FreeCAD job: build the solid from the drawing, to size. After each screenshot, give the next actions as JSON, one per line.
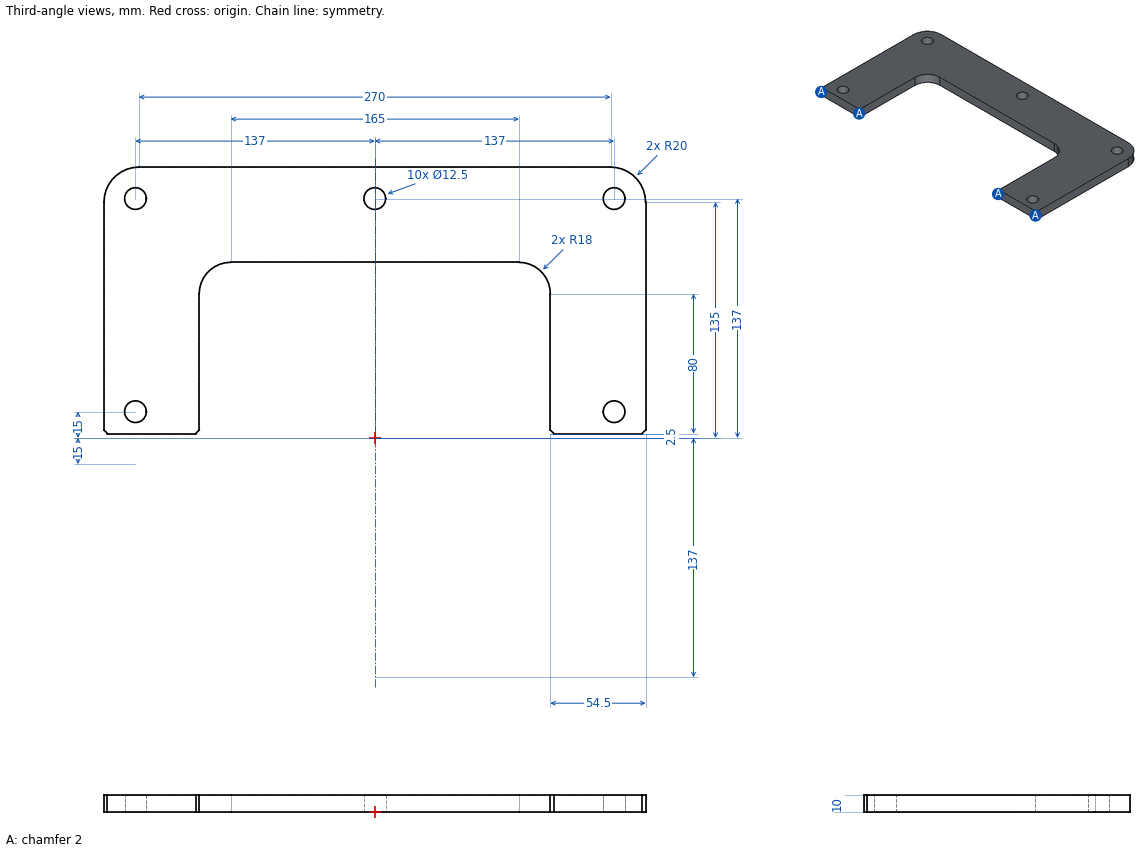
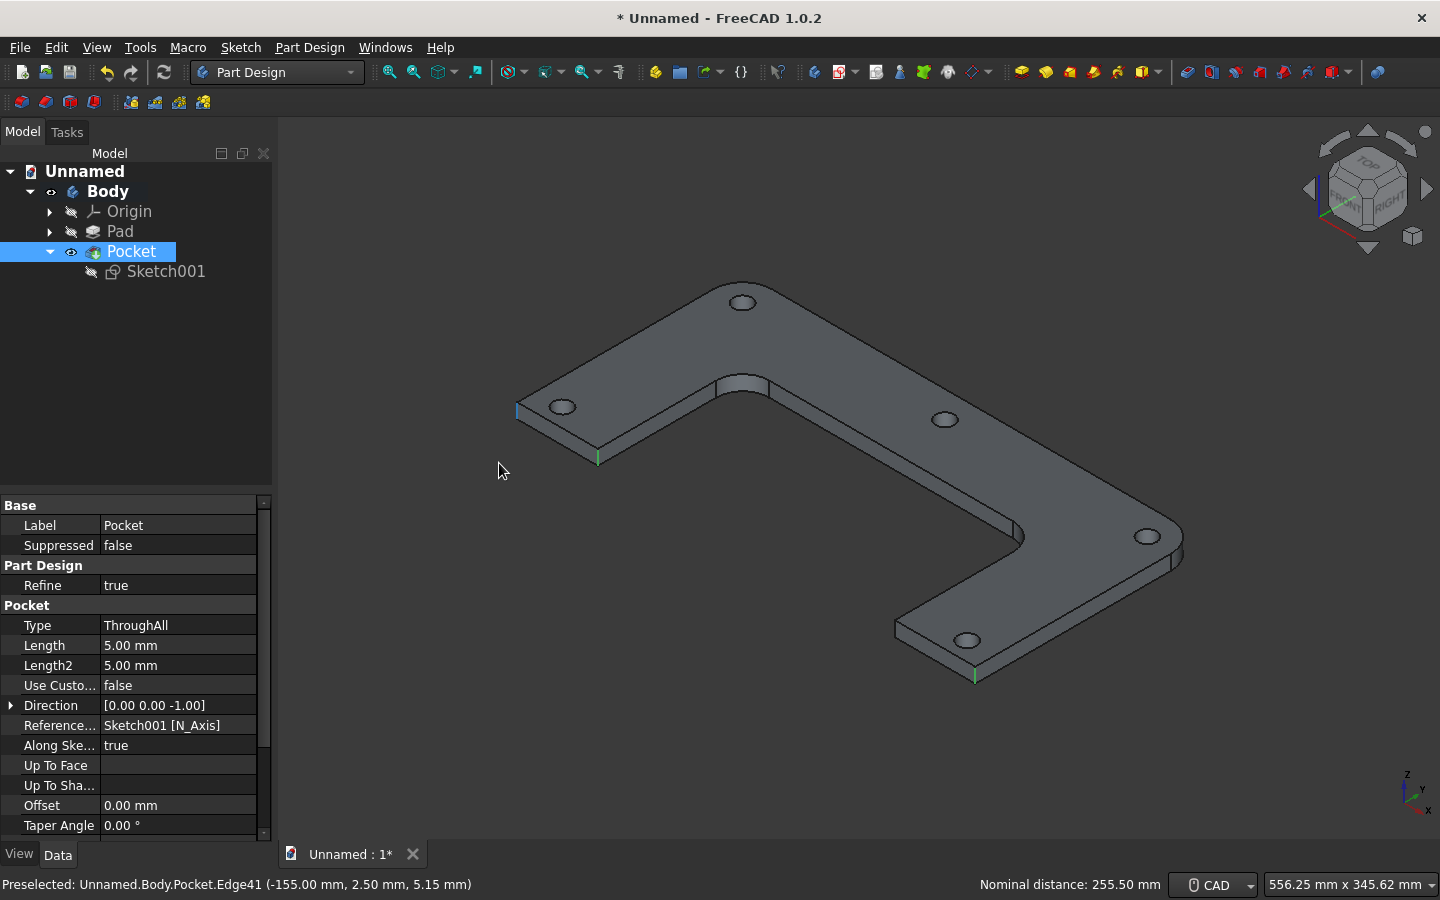
{"action": "scroll", "coordinate": [517, 410], "scroll_direction": "up", "scroll_amount": 4}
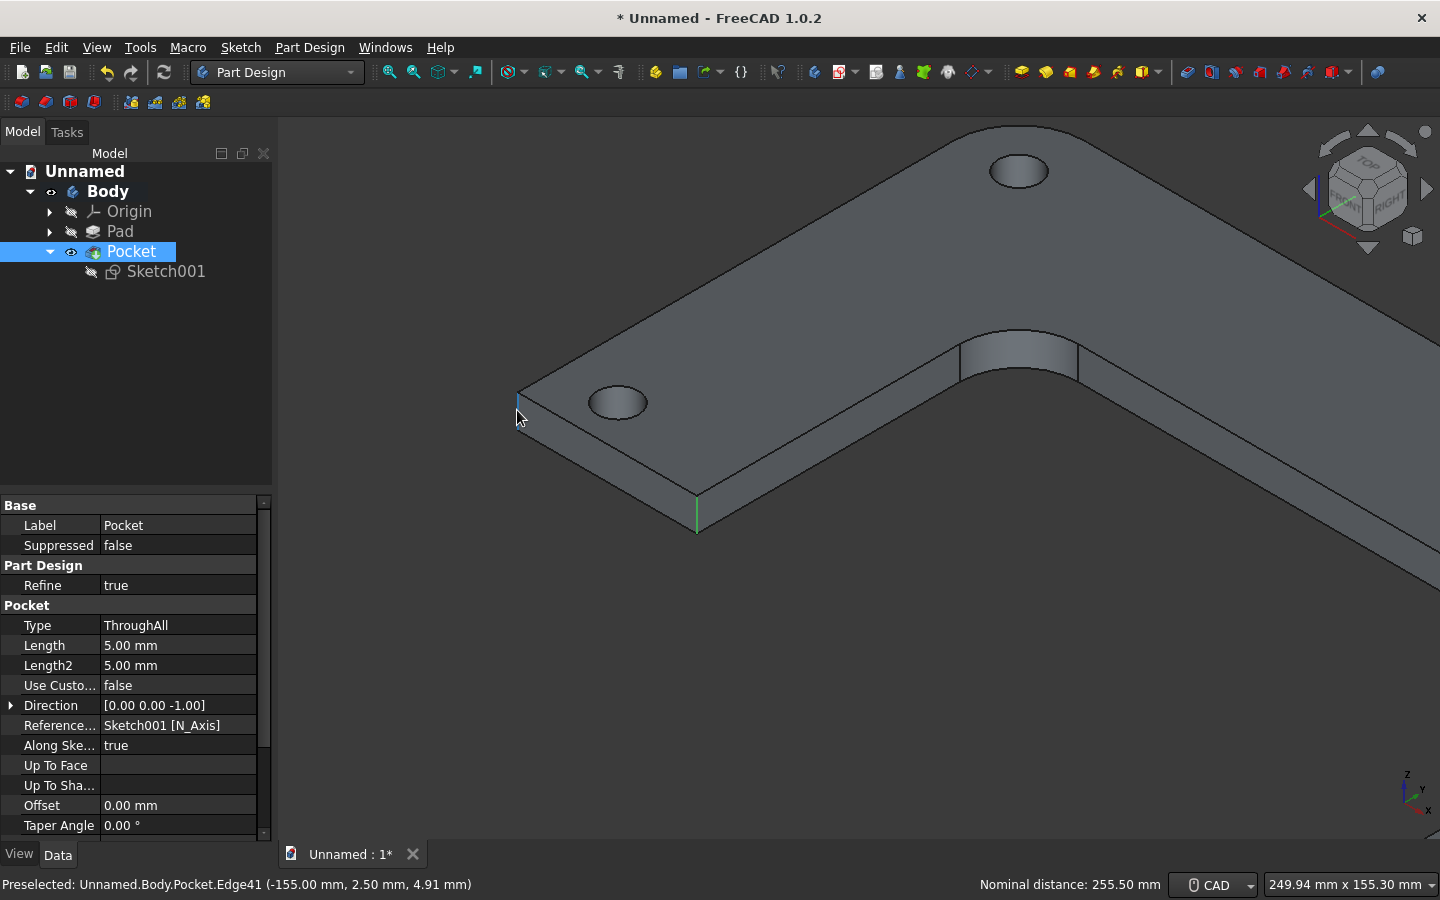
{"action": "key", "text": "v f"}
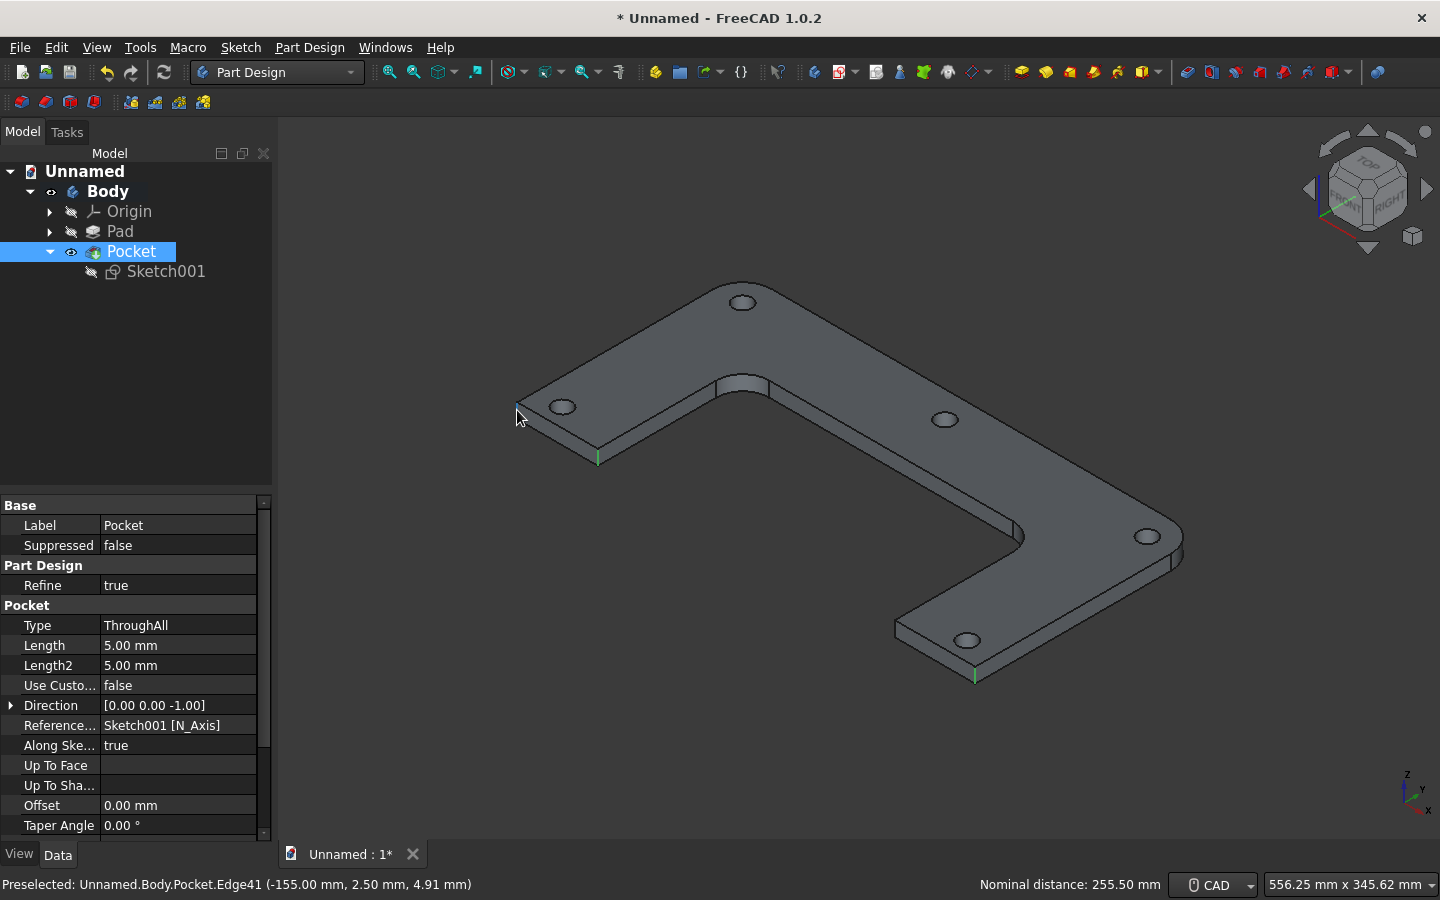
{"action": "key", "text": "2"}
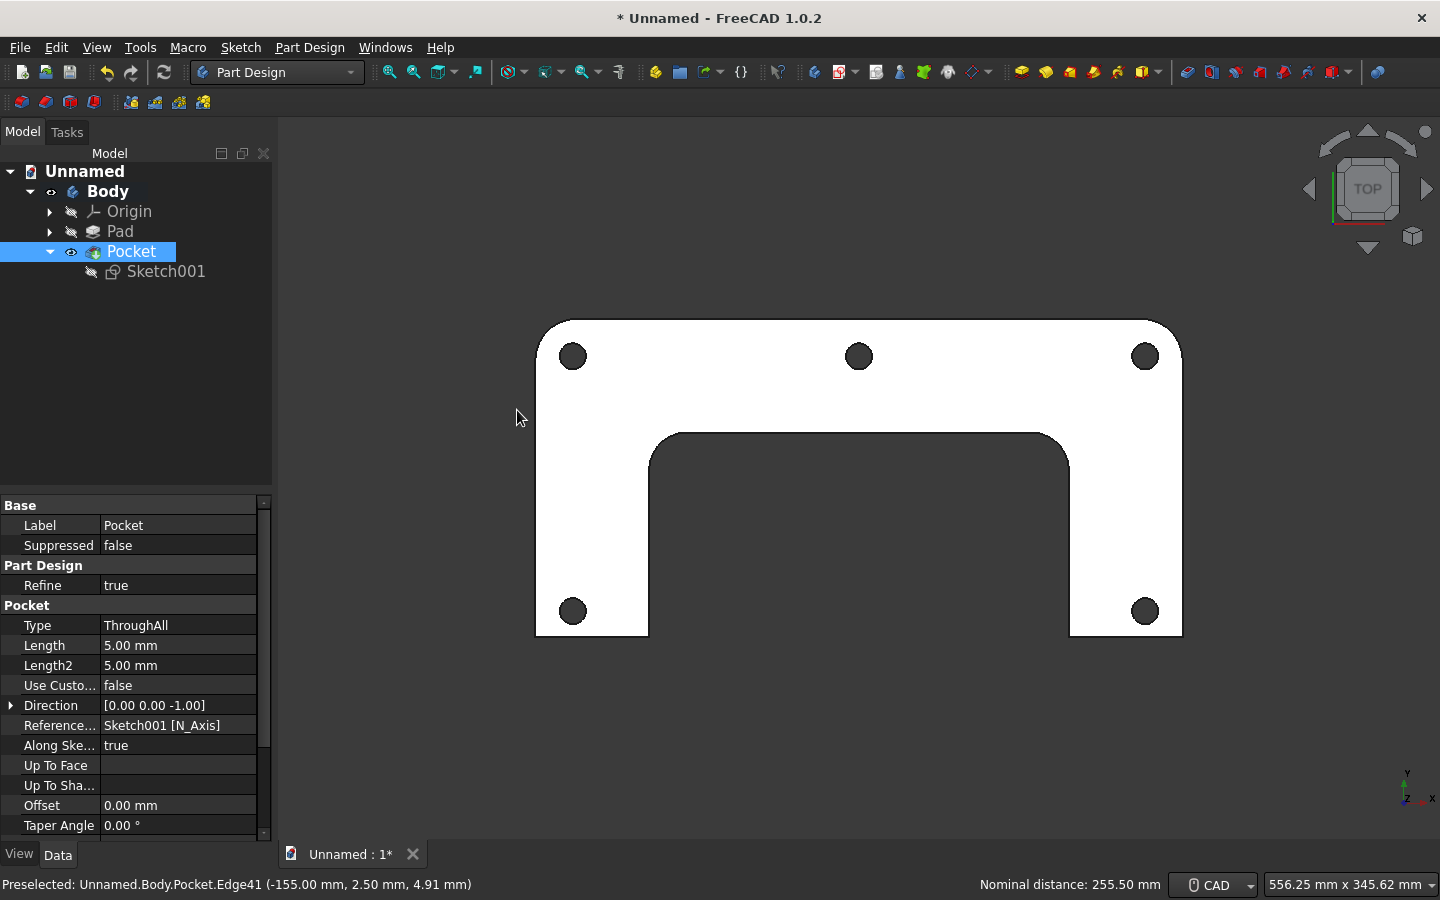
{"action": "scroll", "coordinate": [535, 636], "scroll_direction": "up", "scroll_amount": 4}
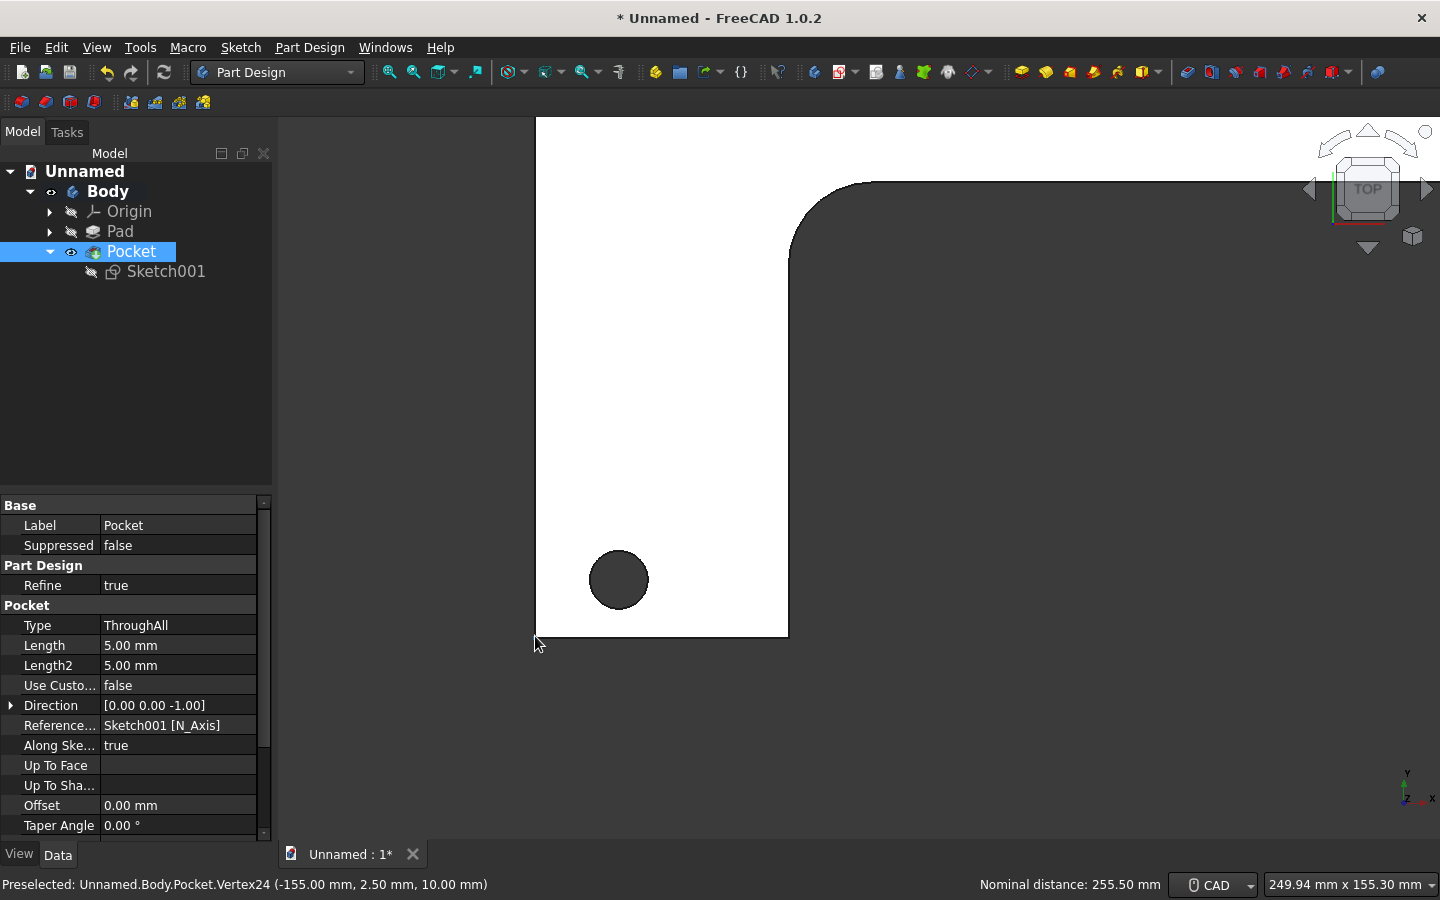
{"action": "key", "text": "v f"}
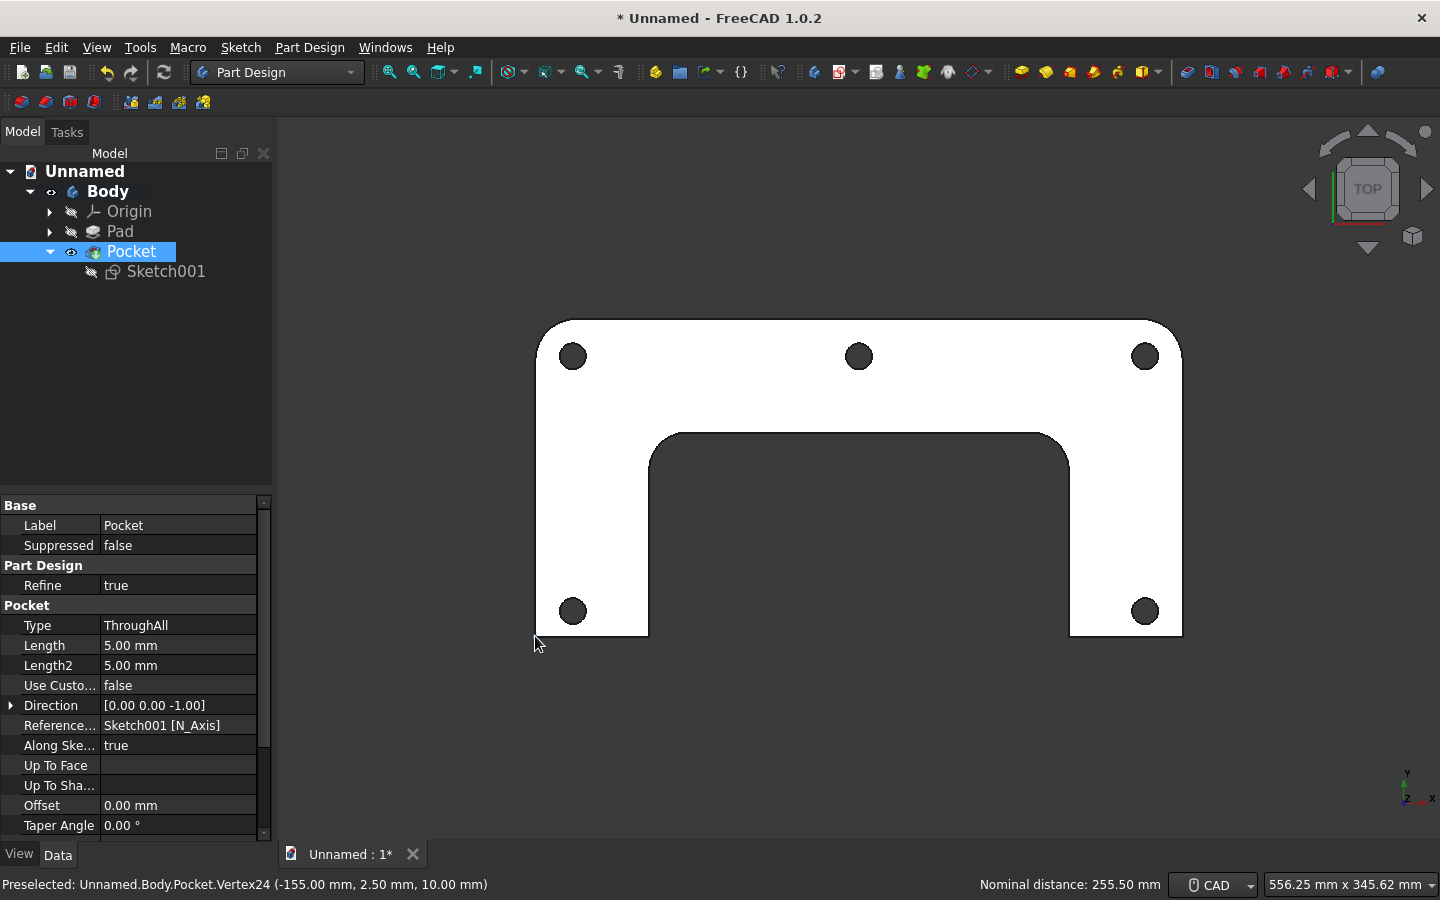
{"action": "key", "text": "1"}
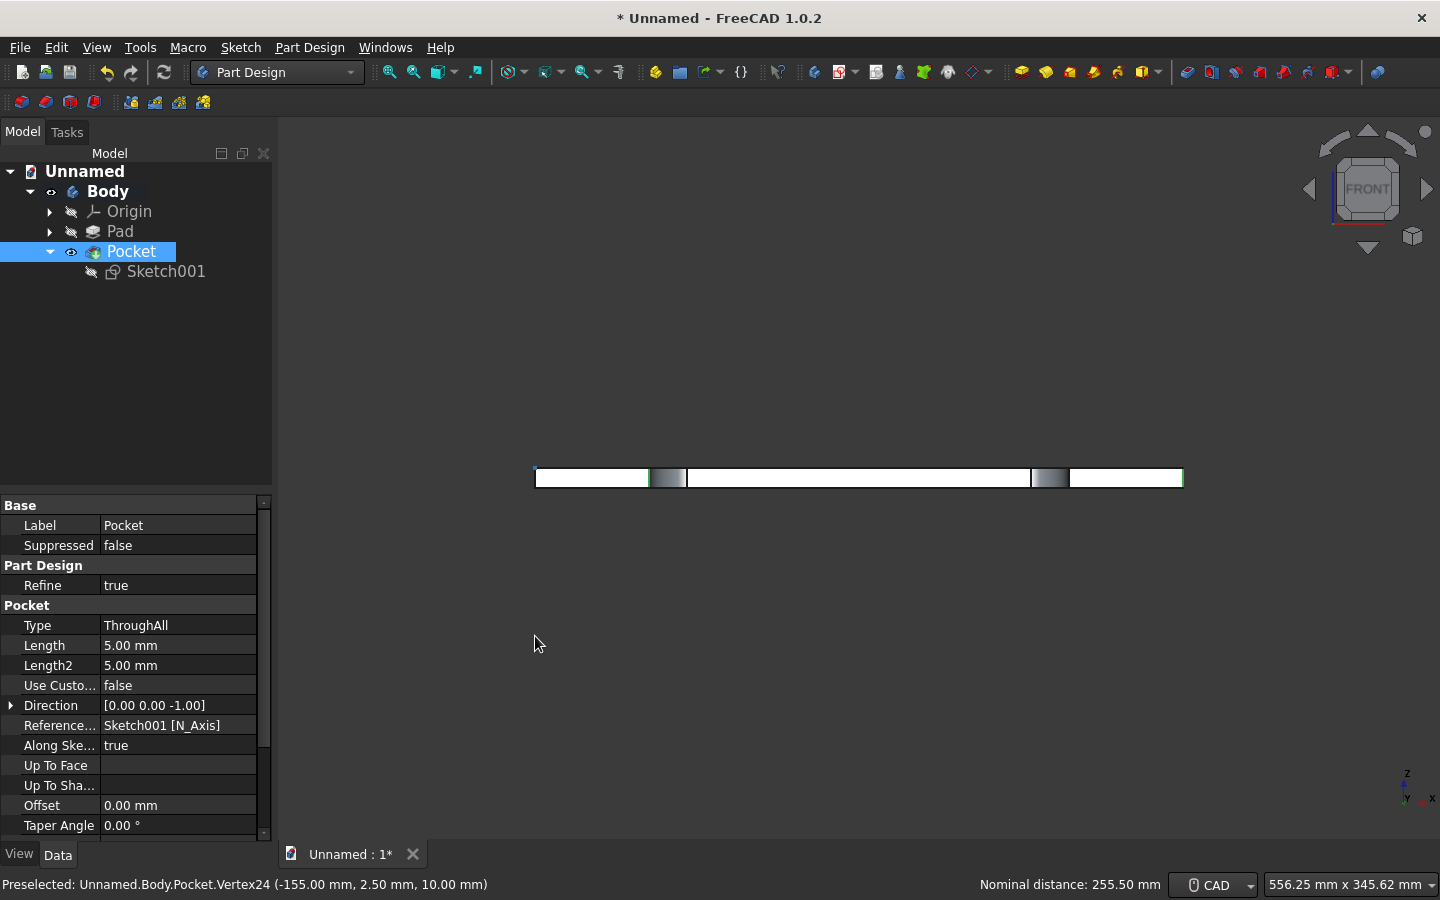
{"action": "left_click", "coordinate": [535, 477], "text": "ctrl"}